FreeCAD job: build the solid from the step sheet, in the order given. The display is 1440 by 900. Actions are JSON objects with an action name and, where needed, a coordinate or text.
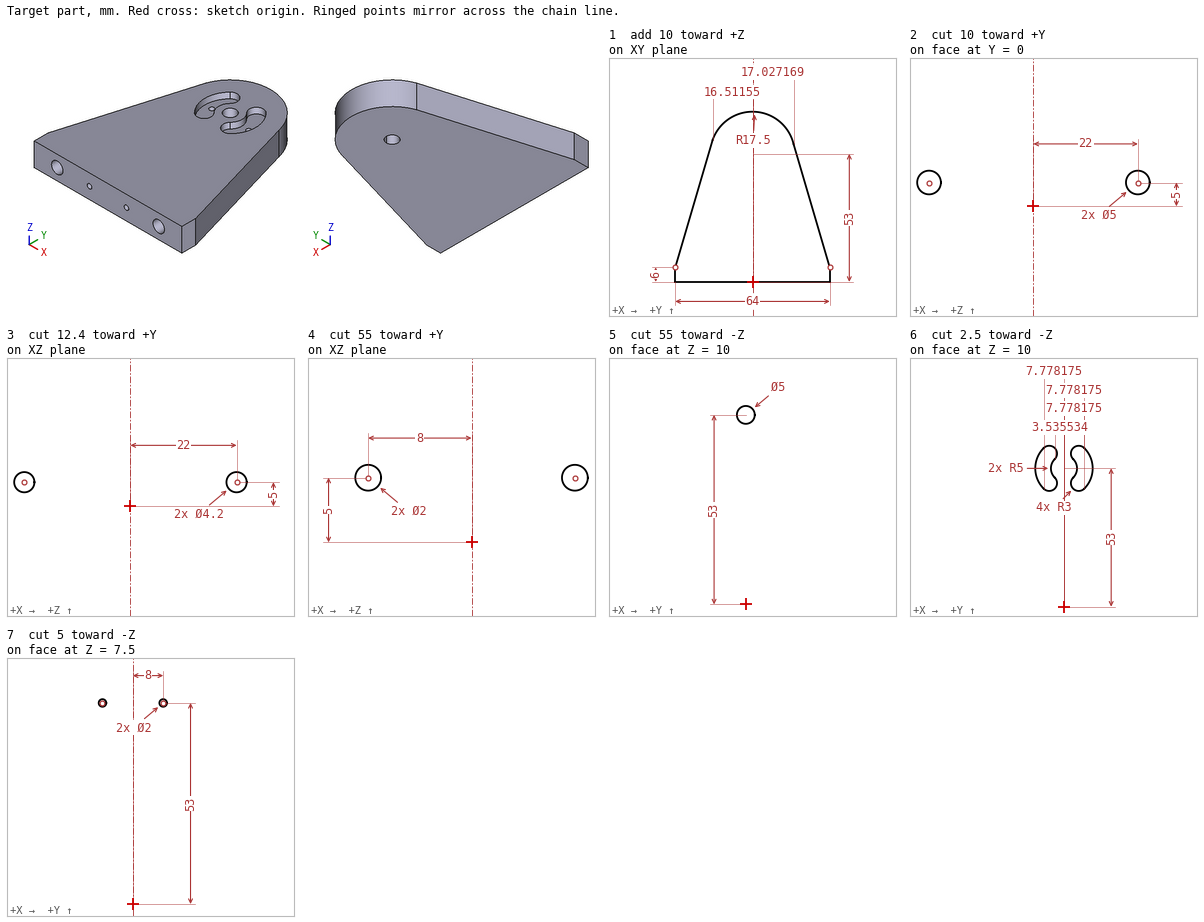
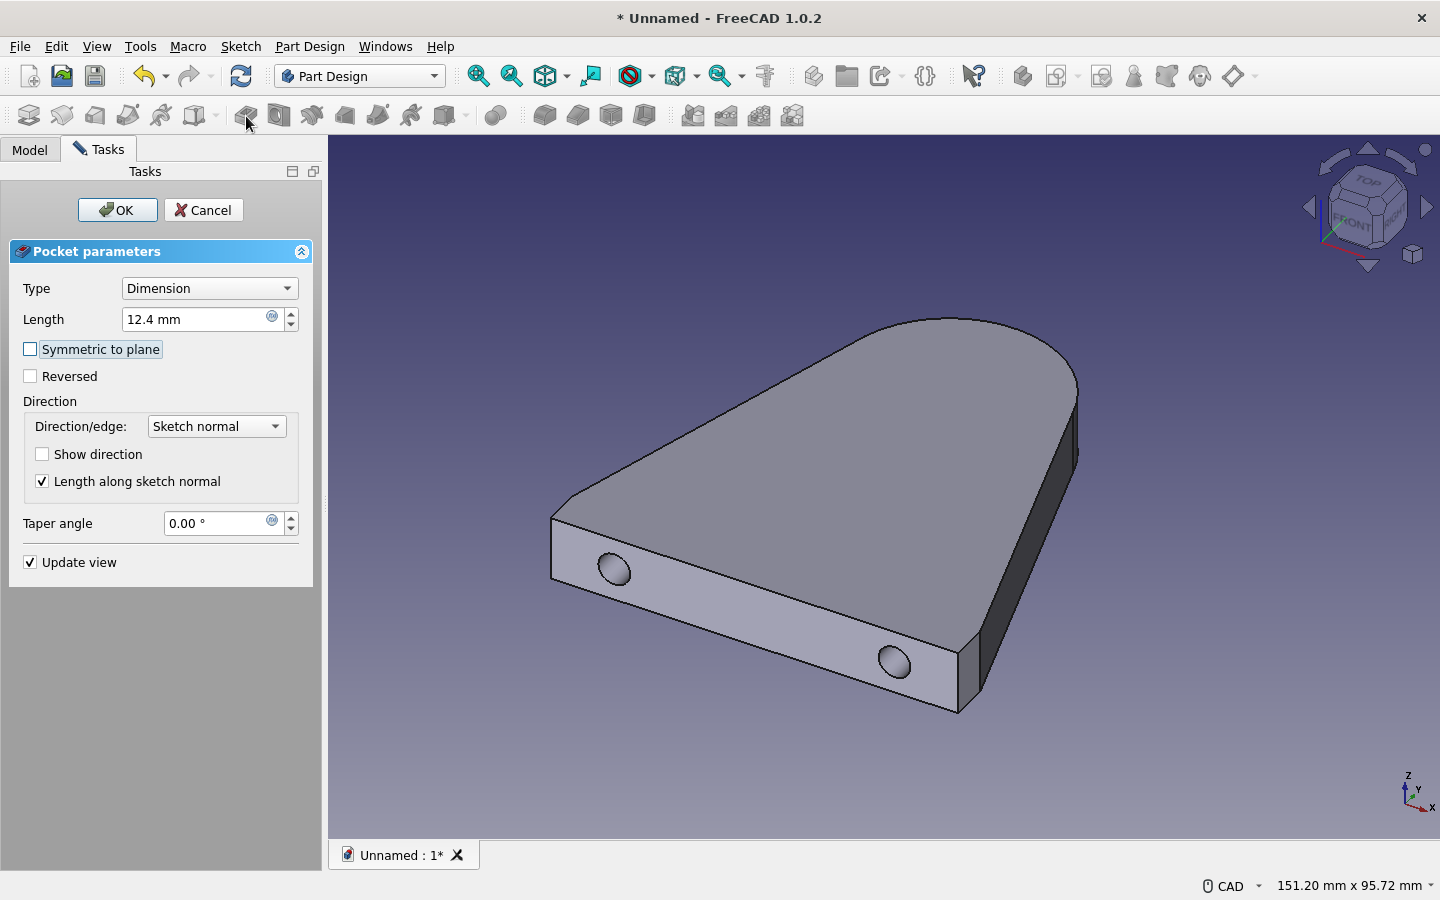
{"action": "left_click", "coordinate": [118, 210]}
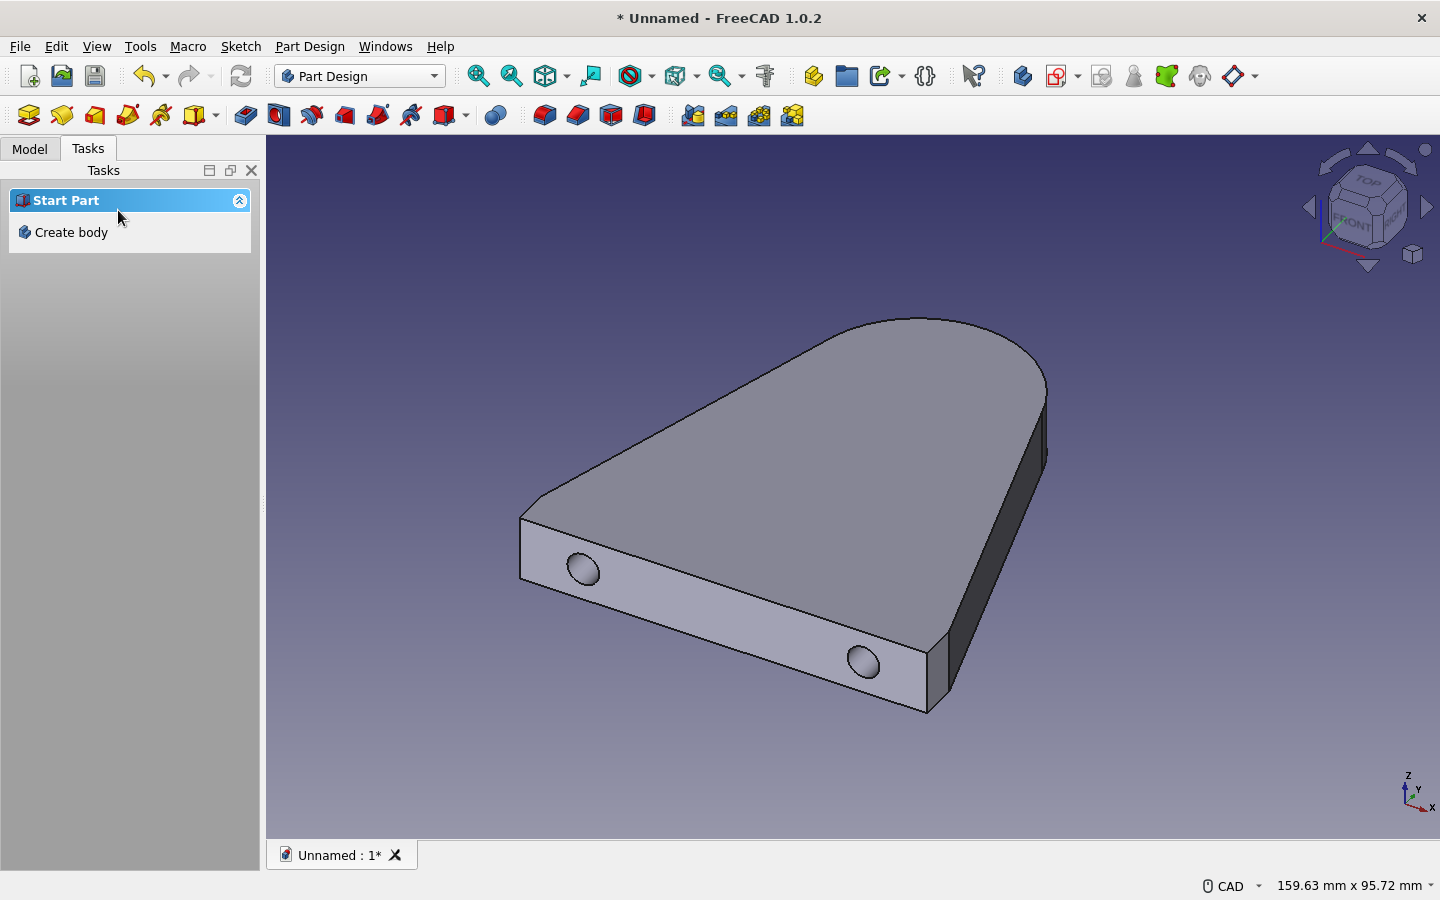
{"action": "left_click", "coordinate": [1056, 76]}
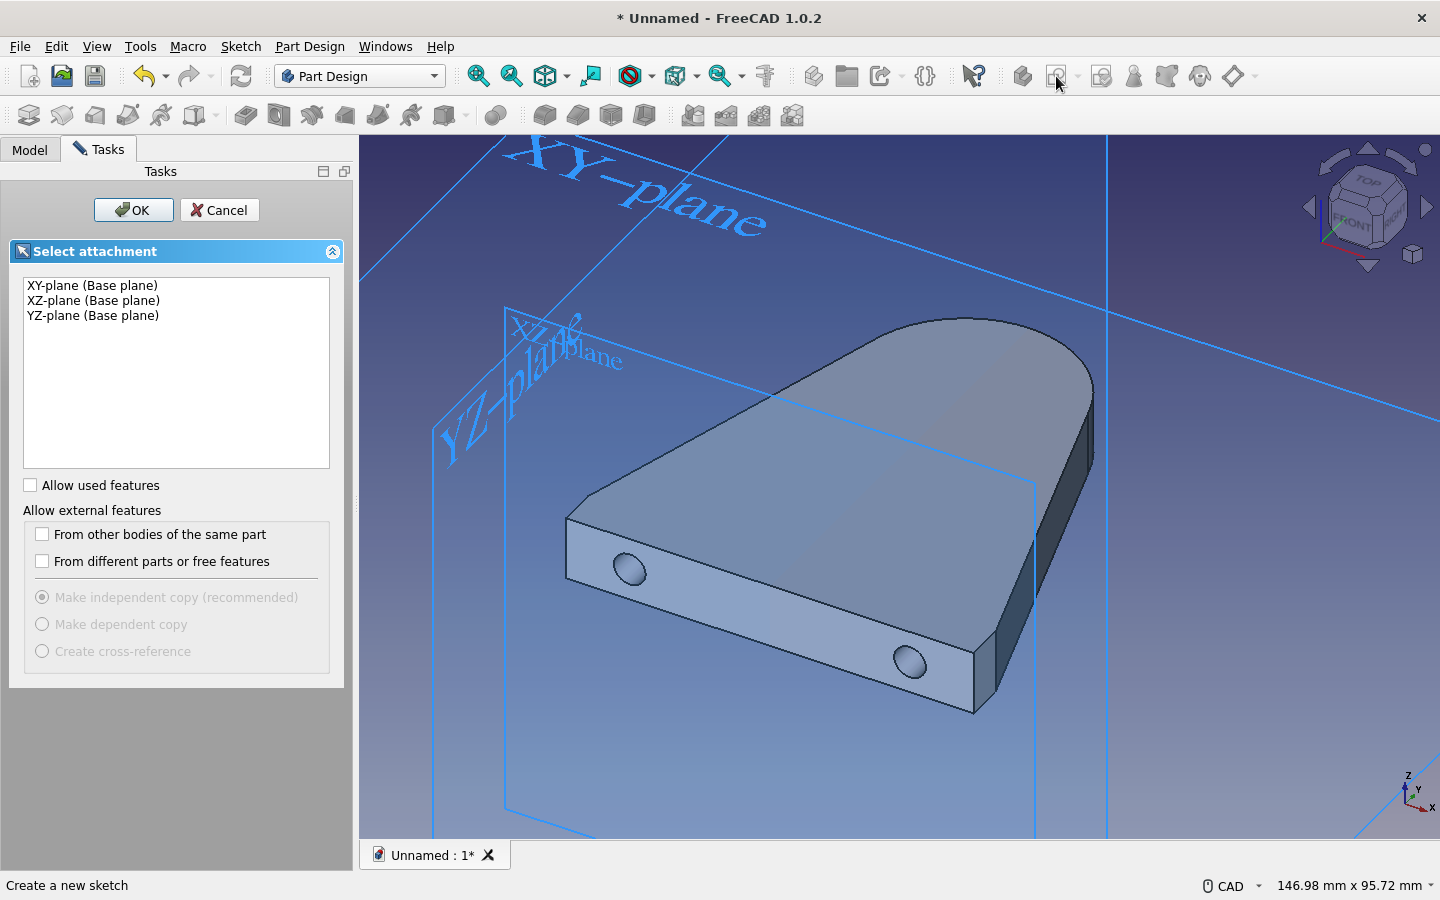
{"action": "left_click", "coordinate": [84, 300]}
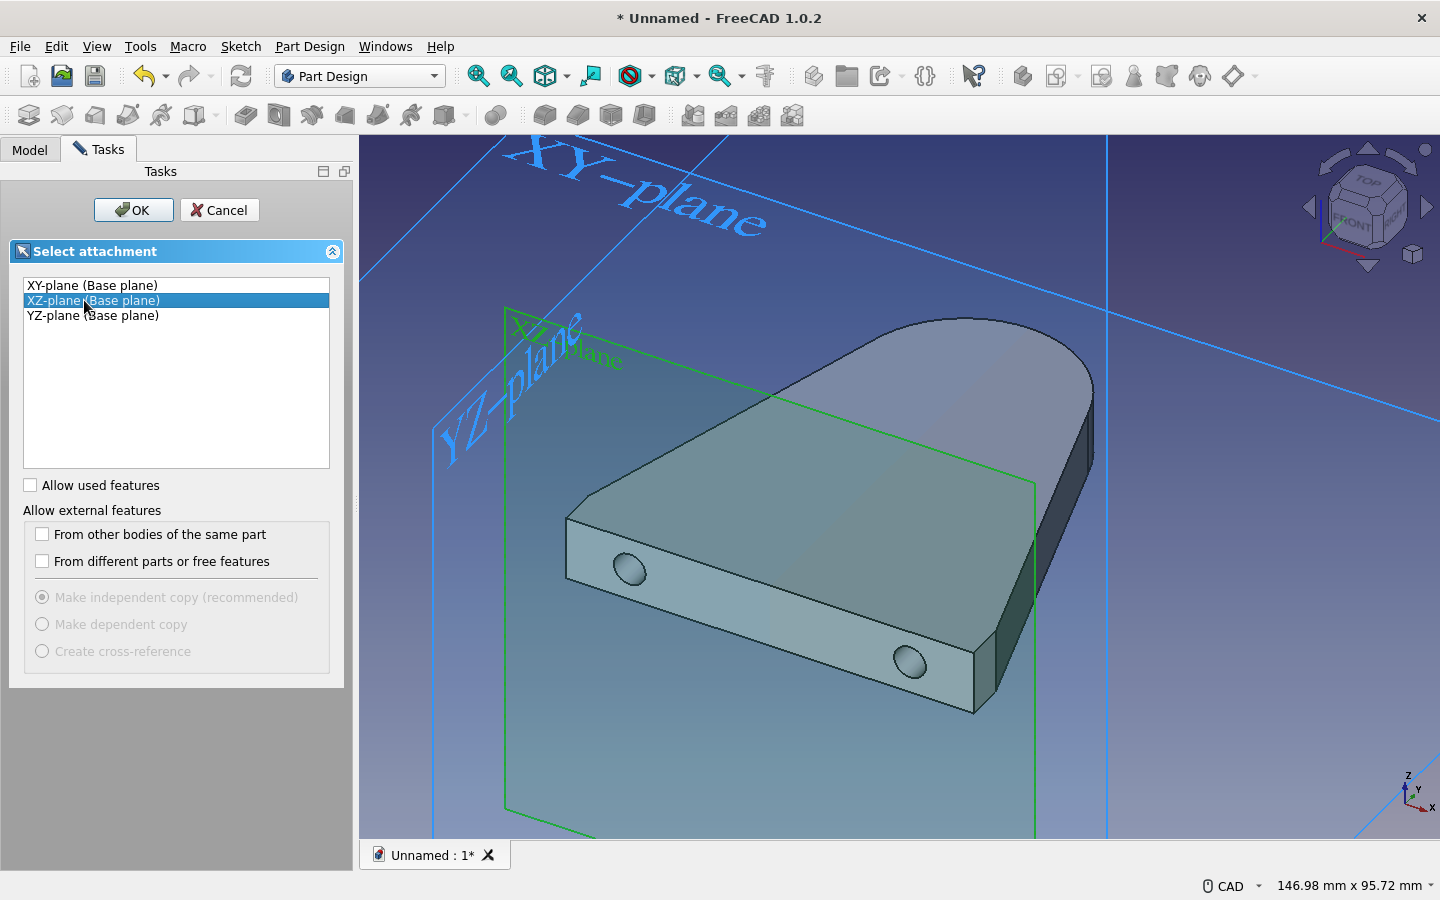
{"action": "left_click", "coordinate": [134, 210]}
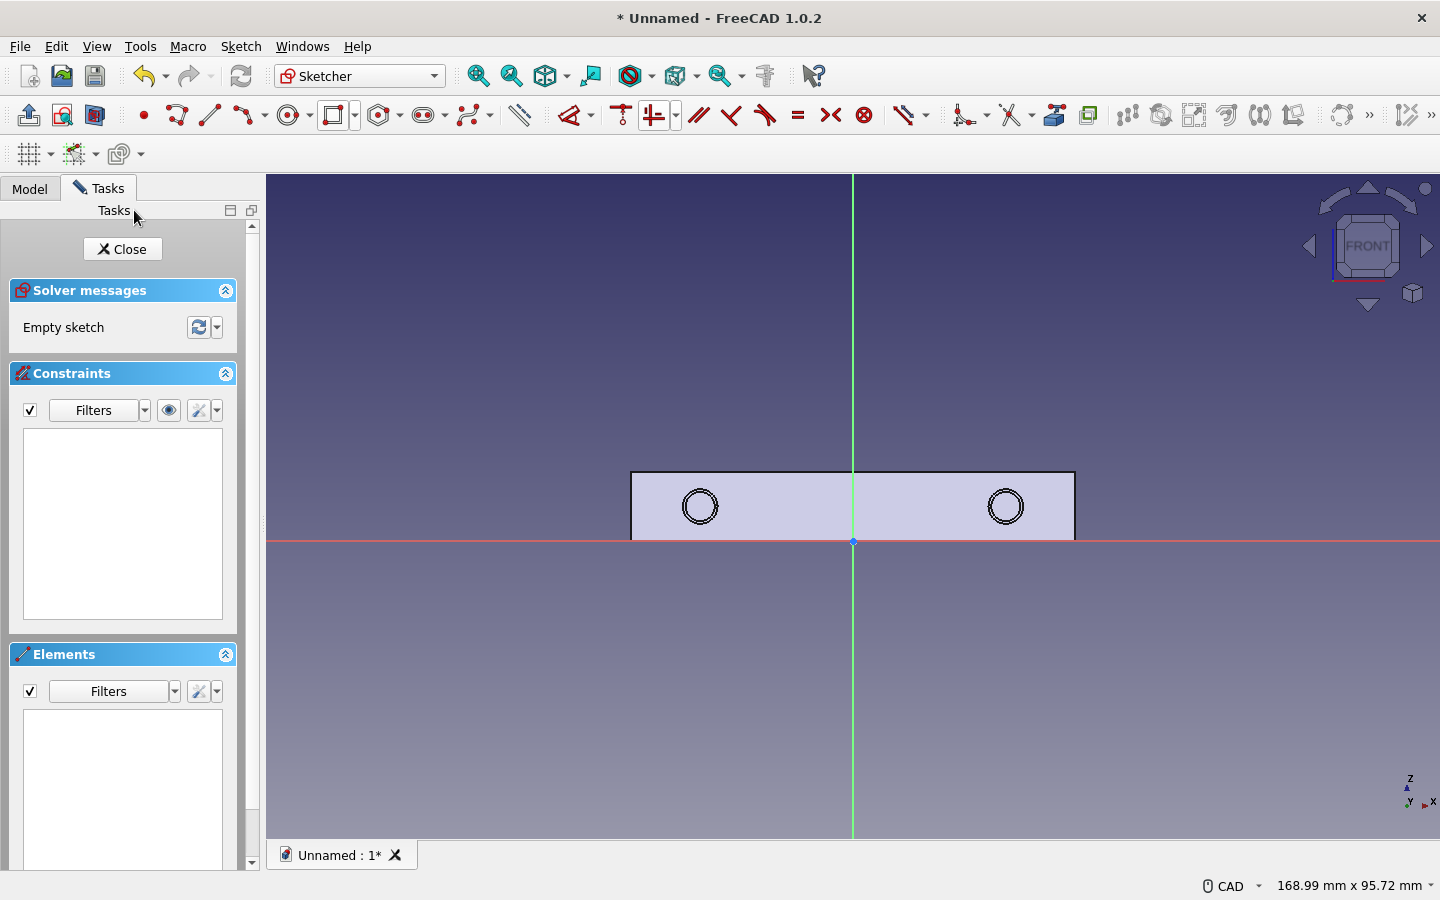
{"action": "scroll", "coordinate": [867, 523], "scroll_direction": "up", "scroll_amount": 9}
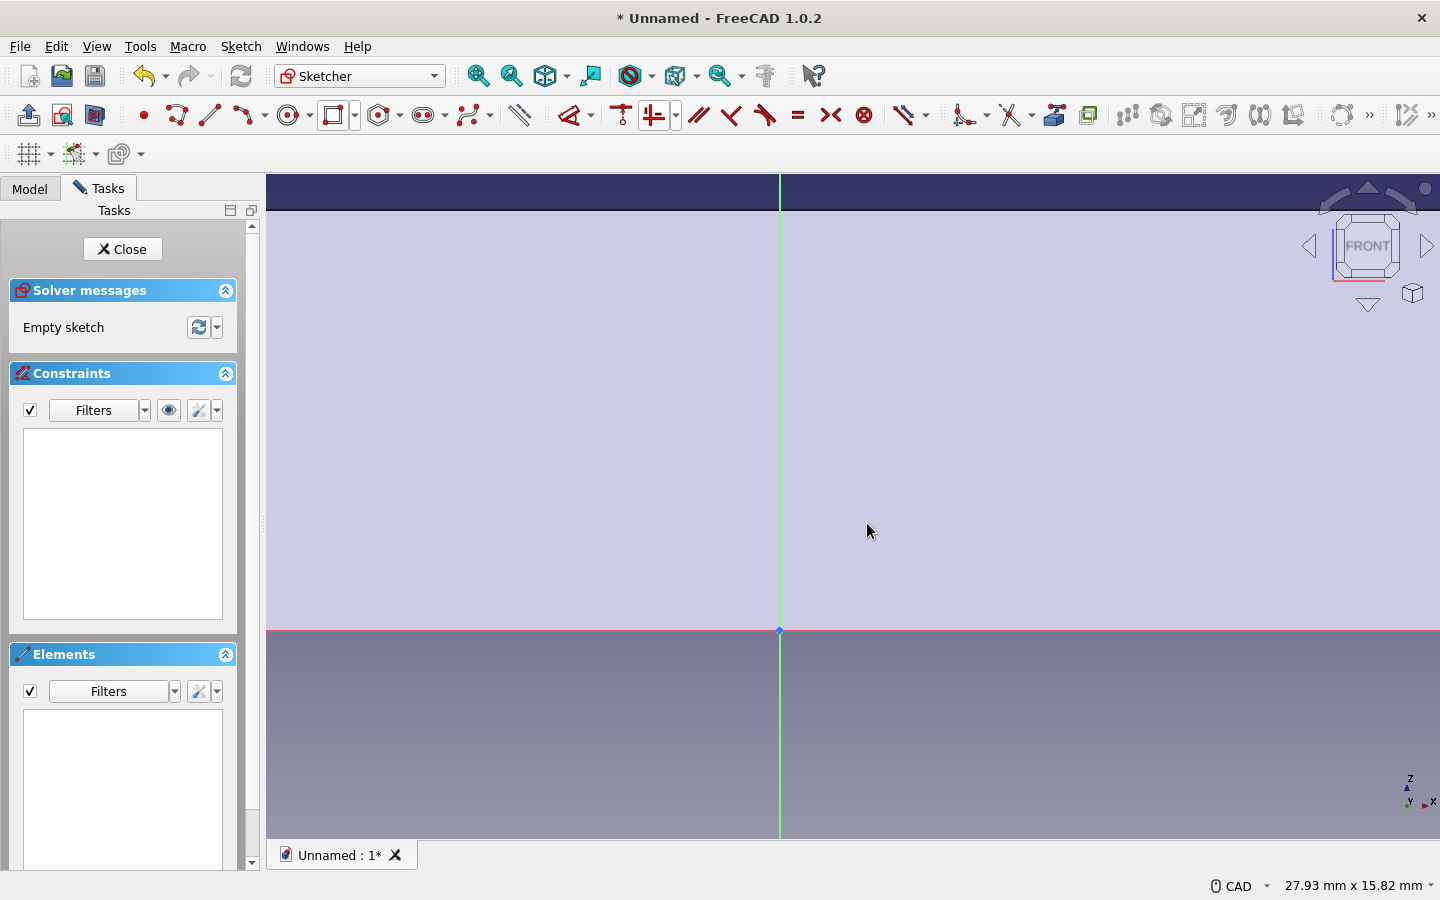
{"action": "left_click", "coordinate": [288, 116]}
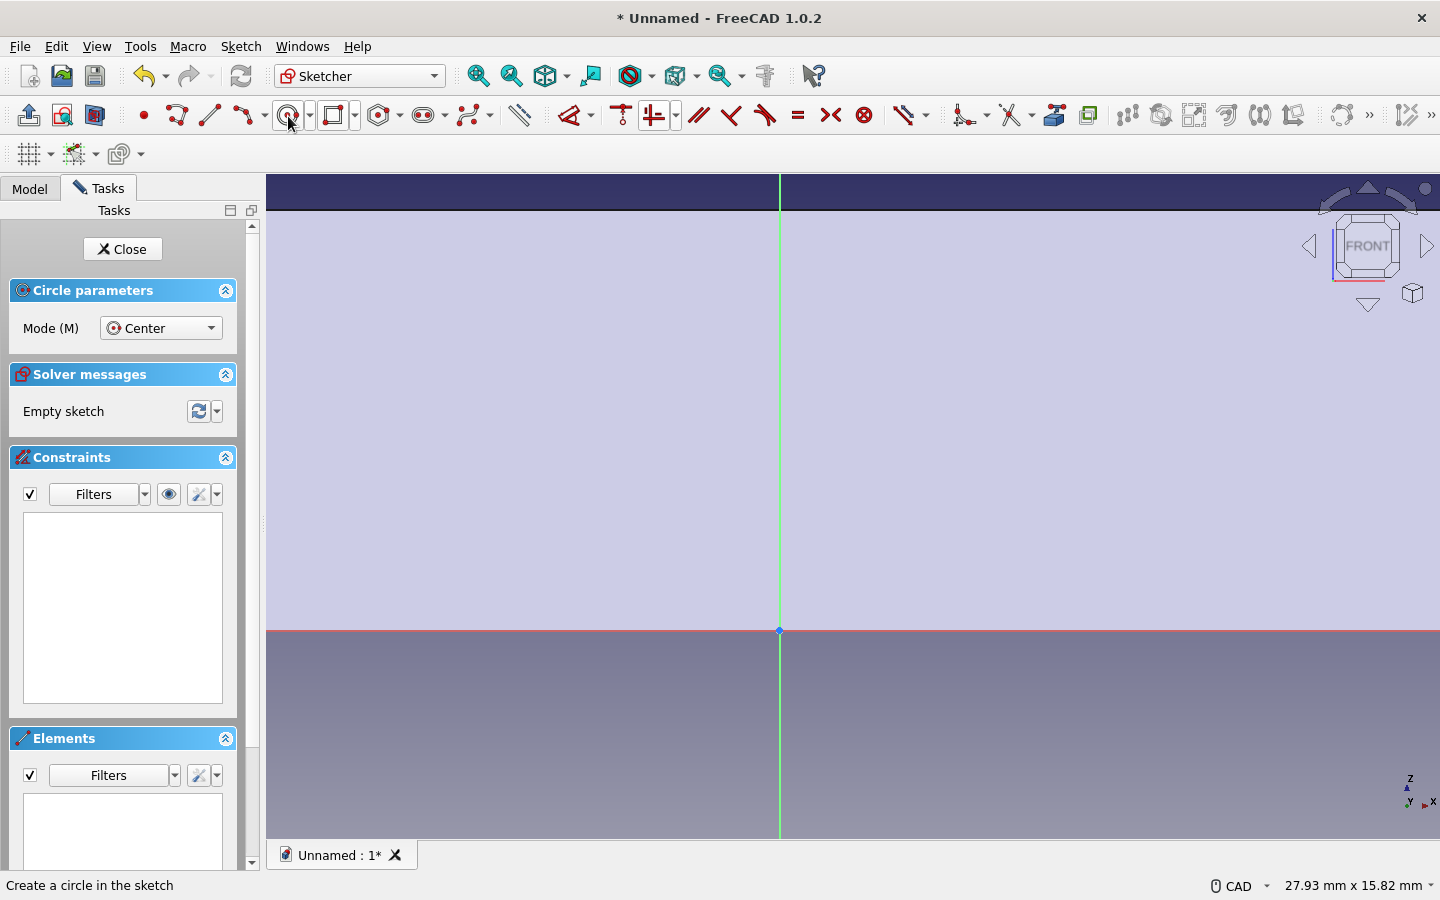
{"action": "left_click", "coordinate": [443, 421]}
{"action": "mouse_move", "coordinate": [473, 391]}